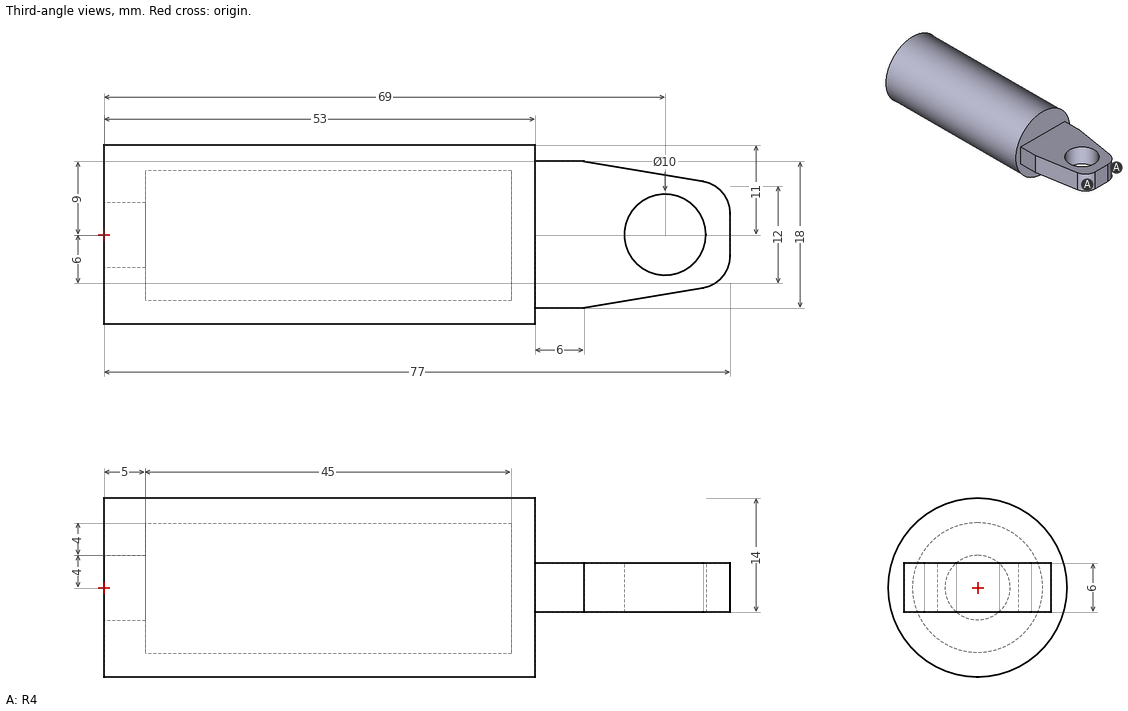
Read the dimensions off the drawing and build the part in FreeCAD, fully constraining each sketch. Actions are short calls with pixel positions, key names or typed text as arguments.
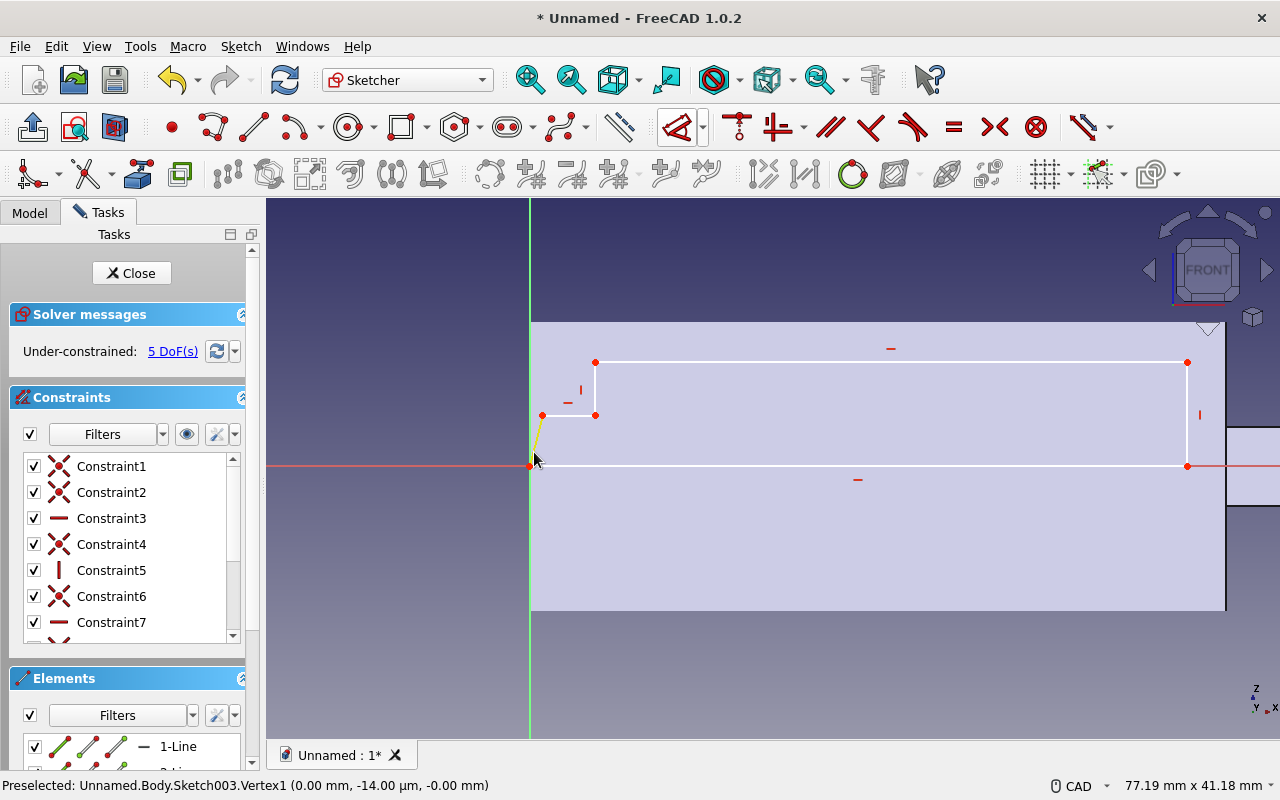
click(534, 451)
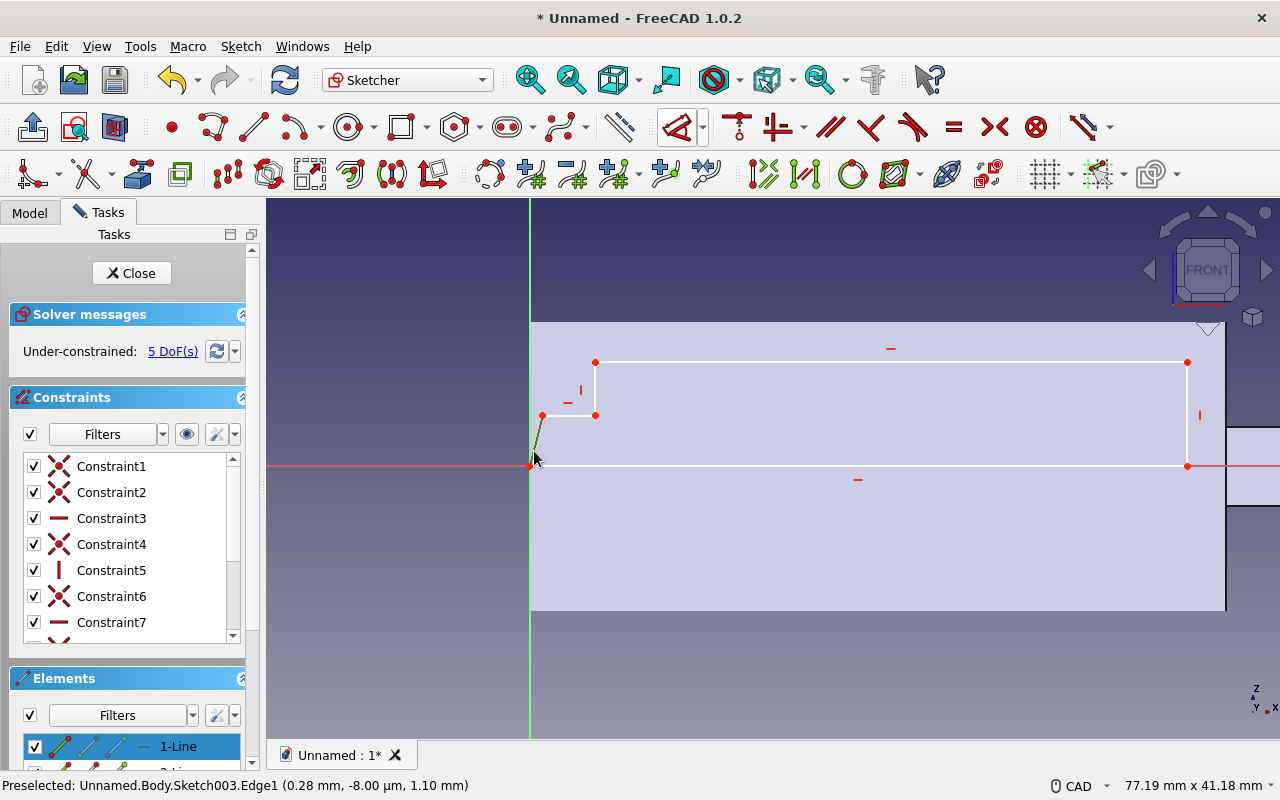
key(v)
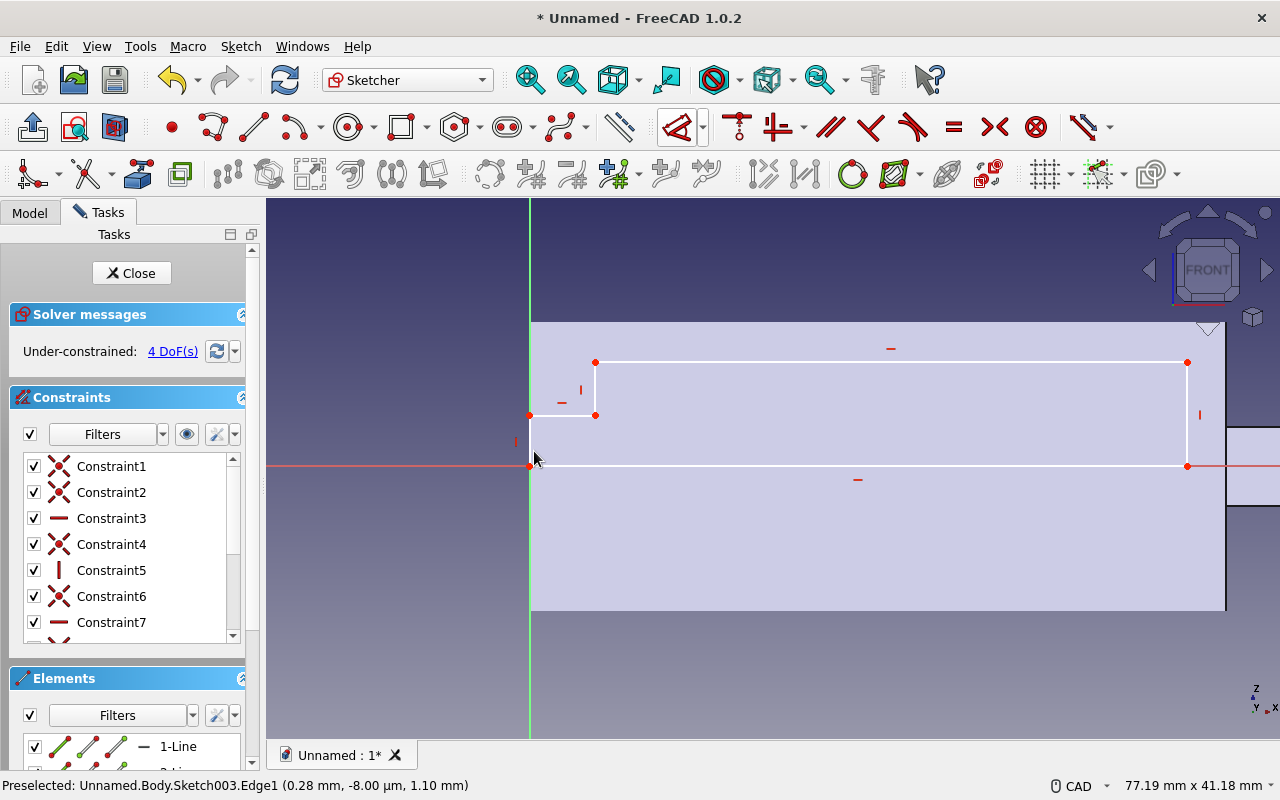
click(530, 451)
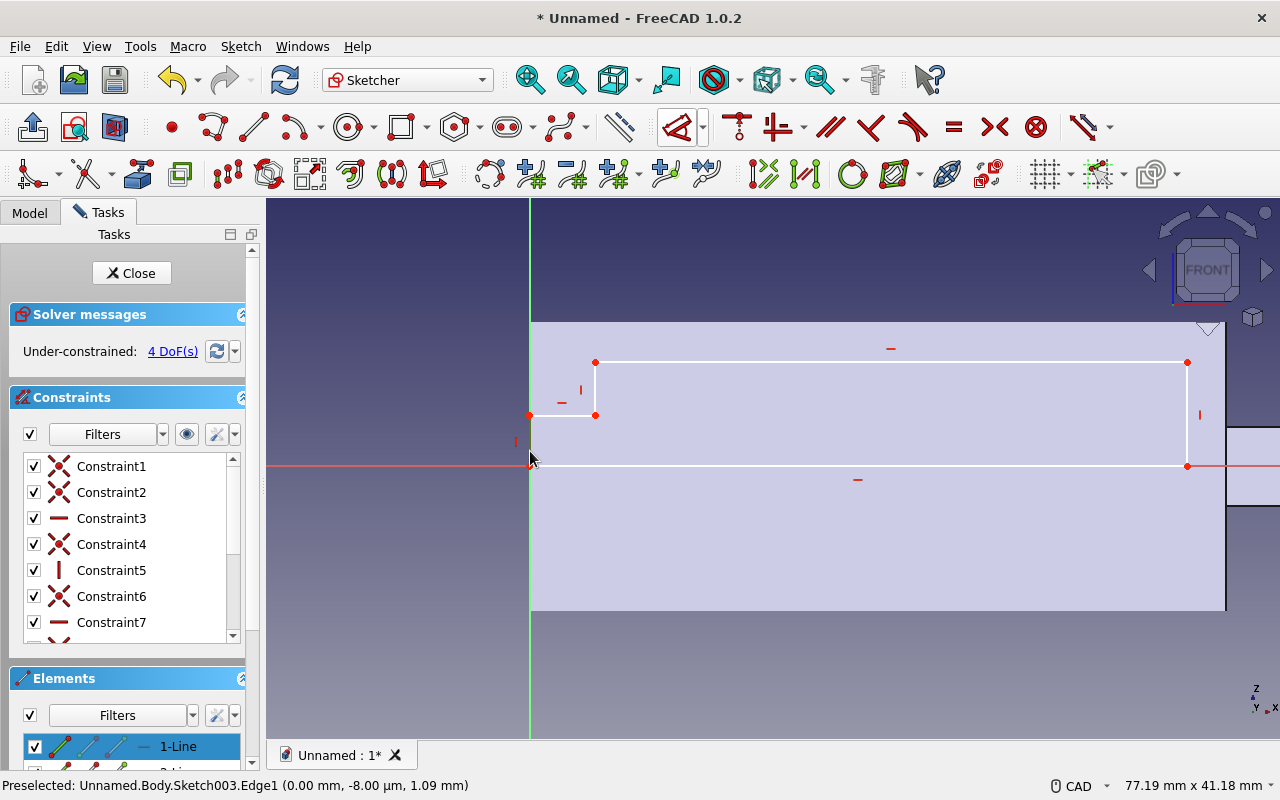
key(i)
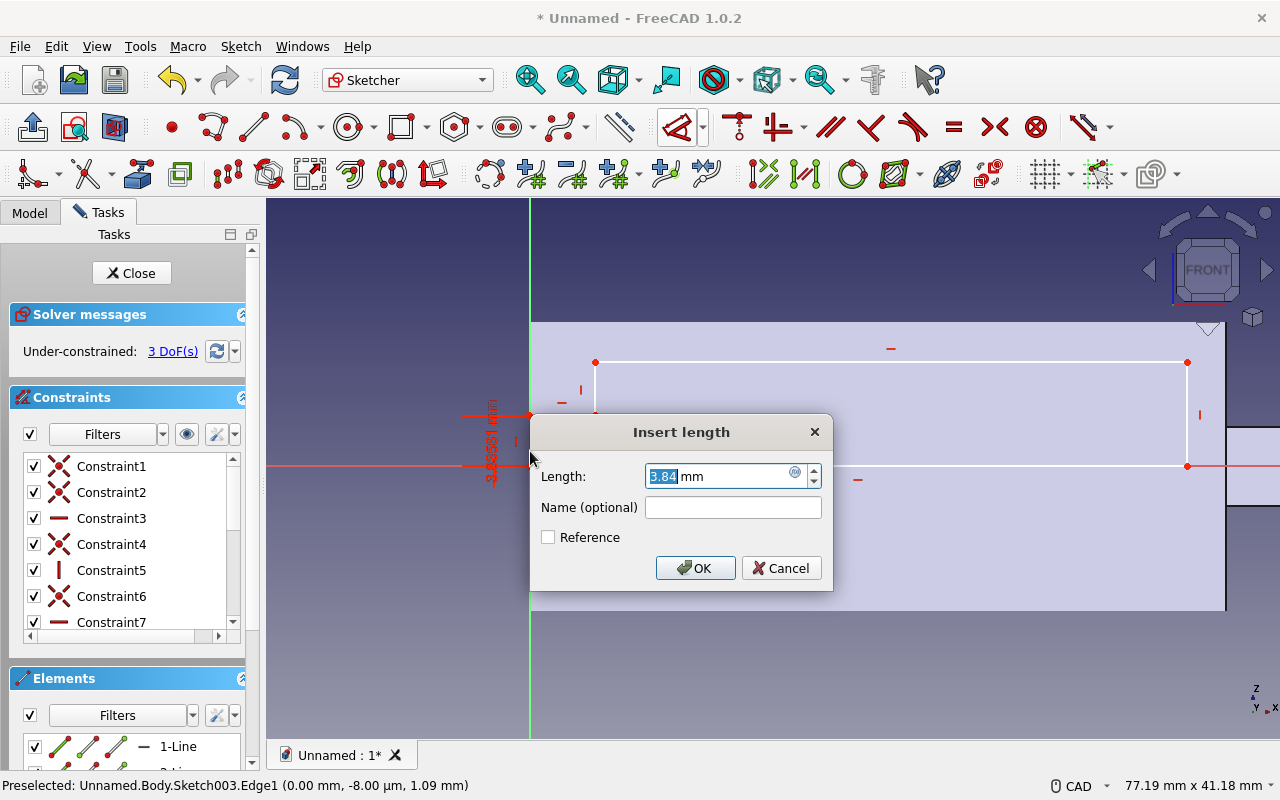
text(4)
key(Return)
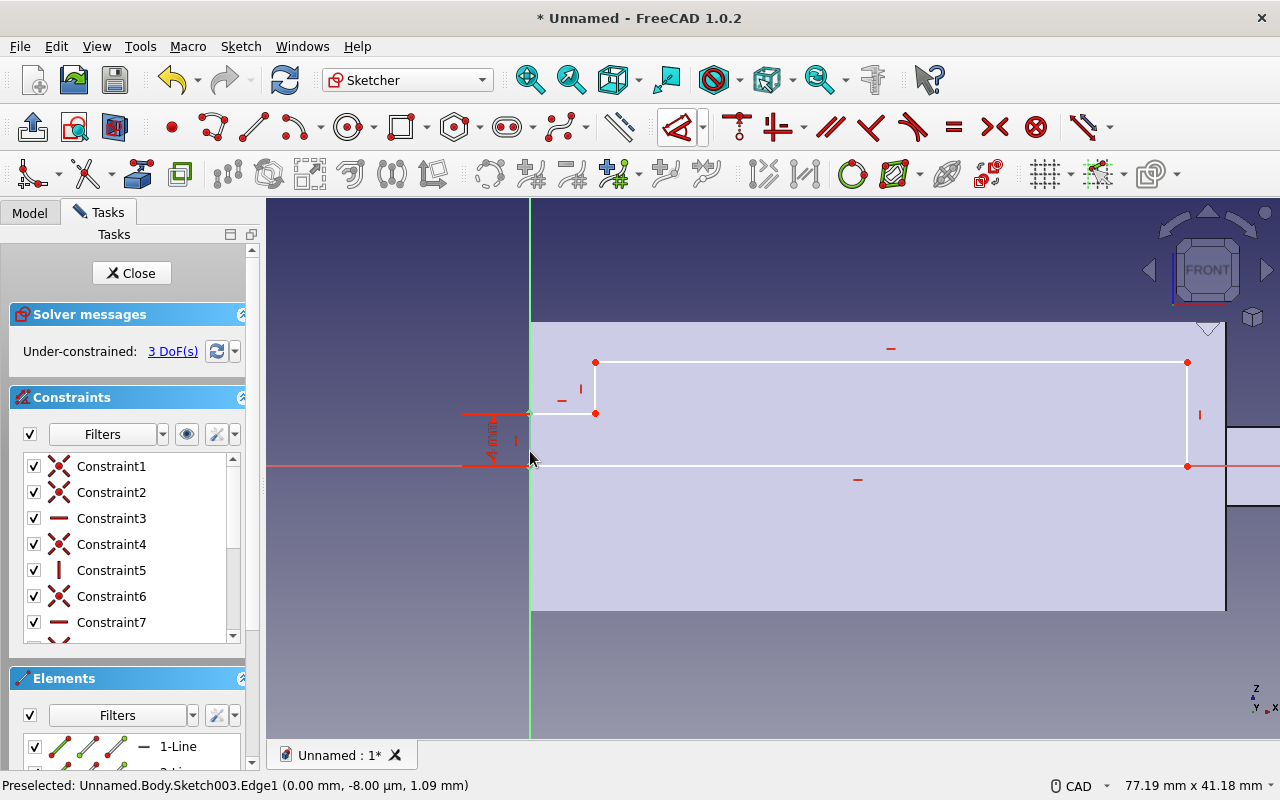
click(549, 414)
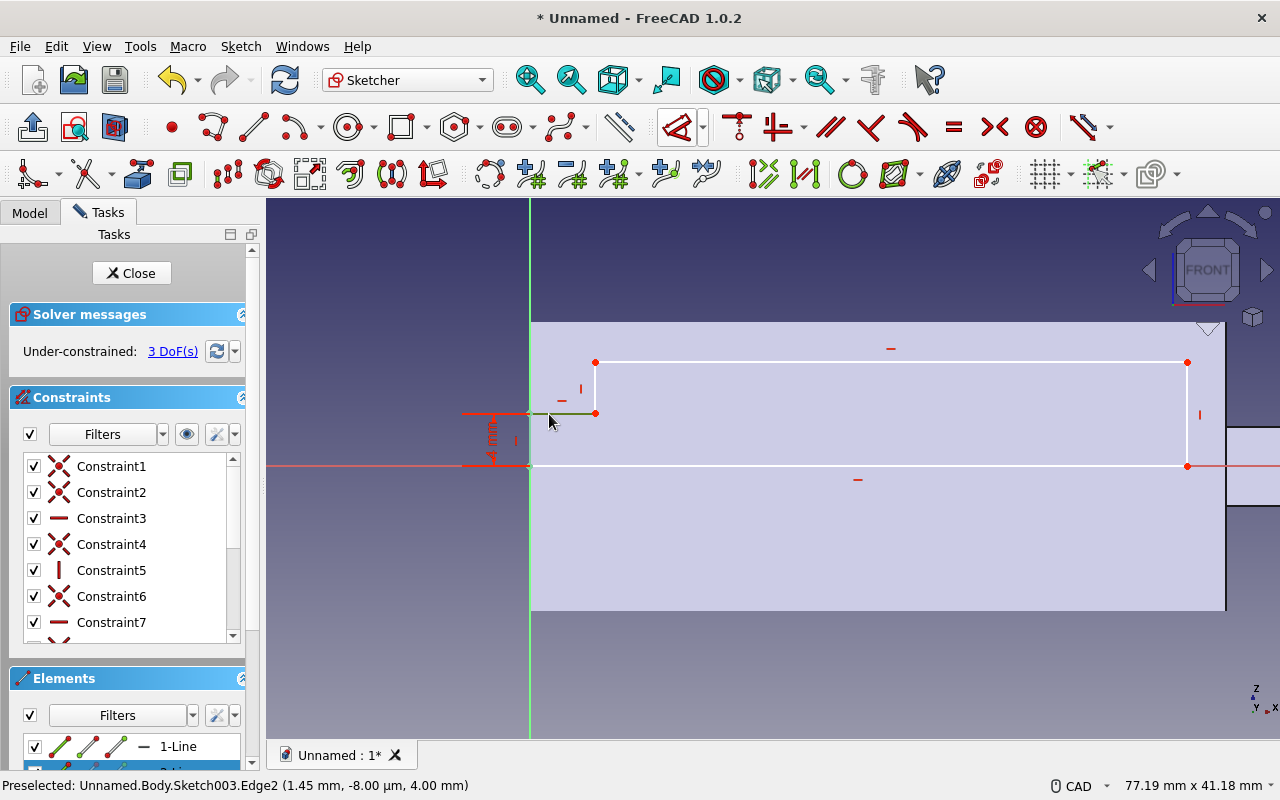
key(l)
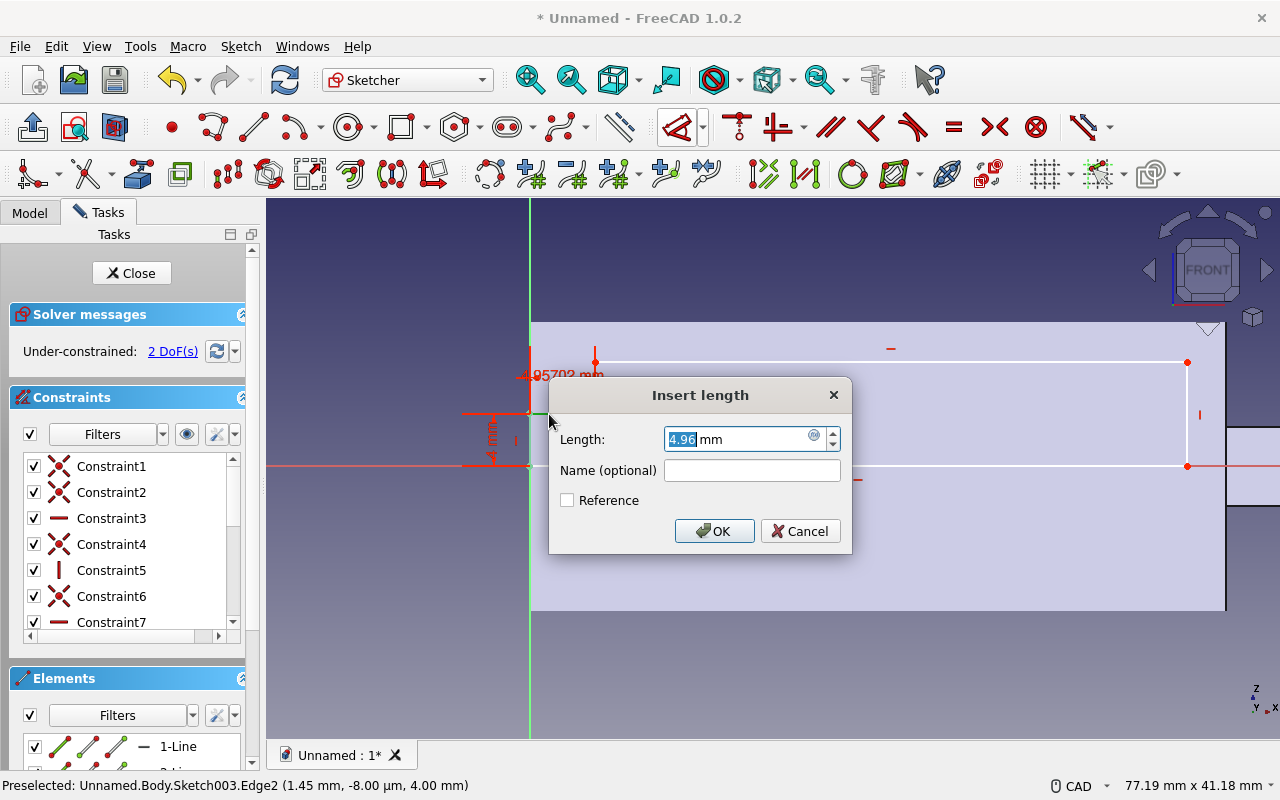
text(5)
key(Return)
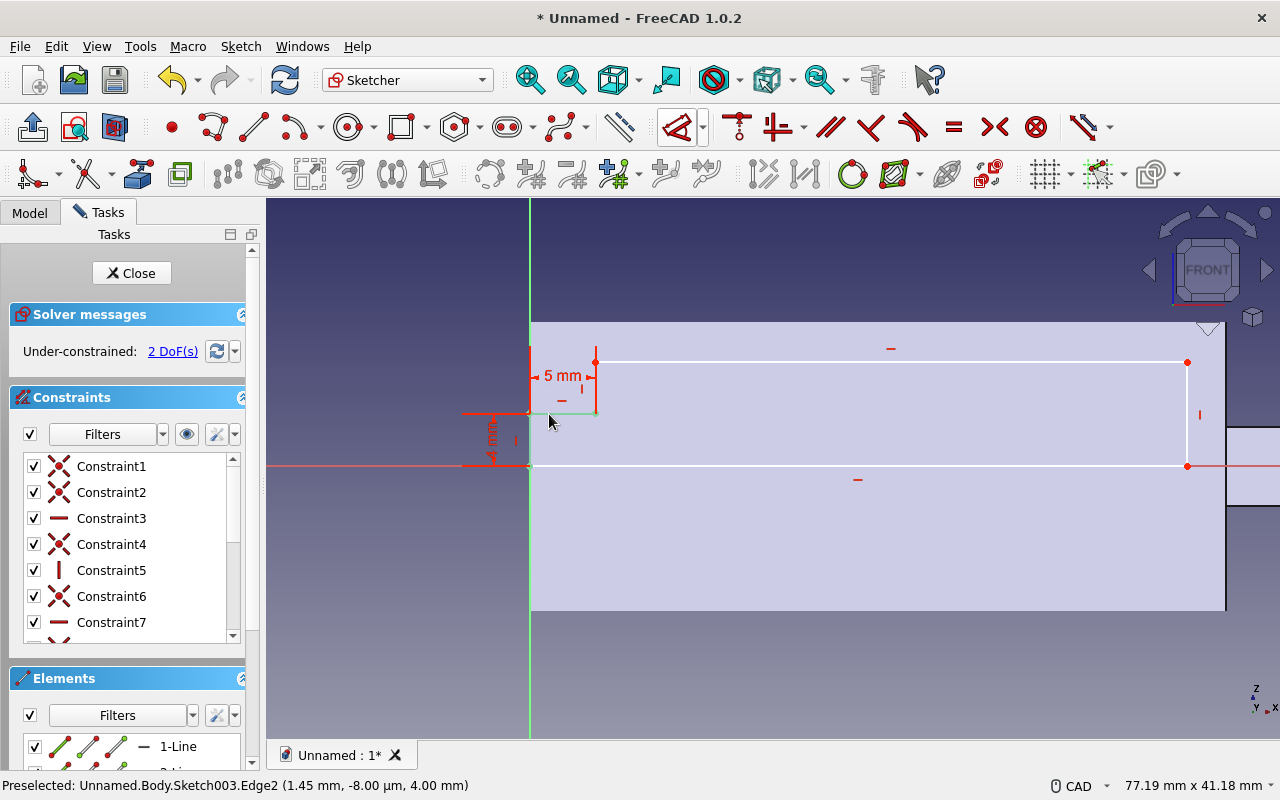
click(596, 398)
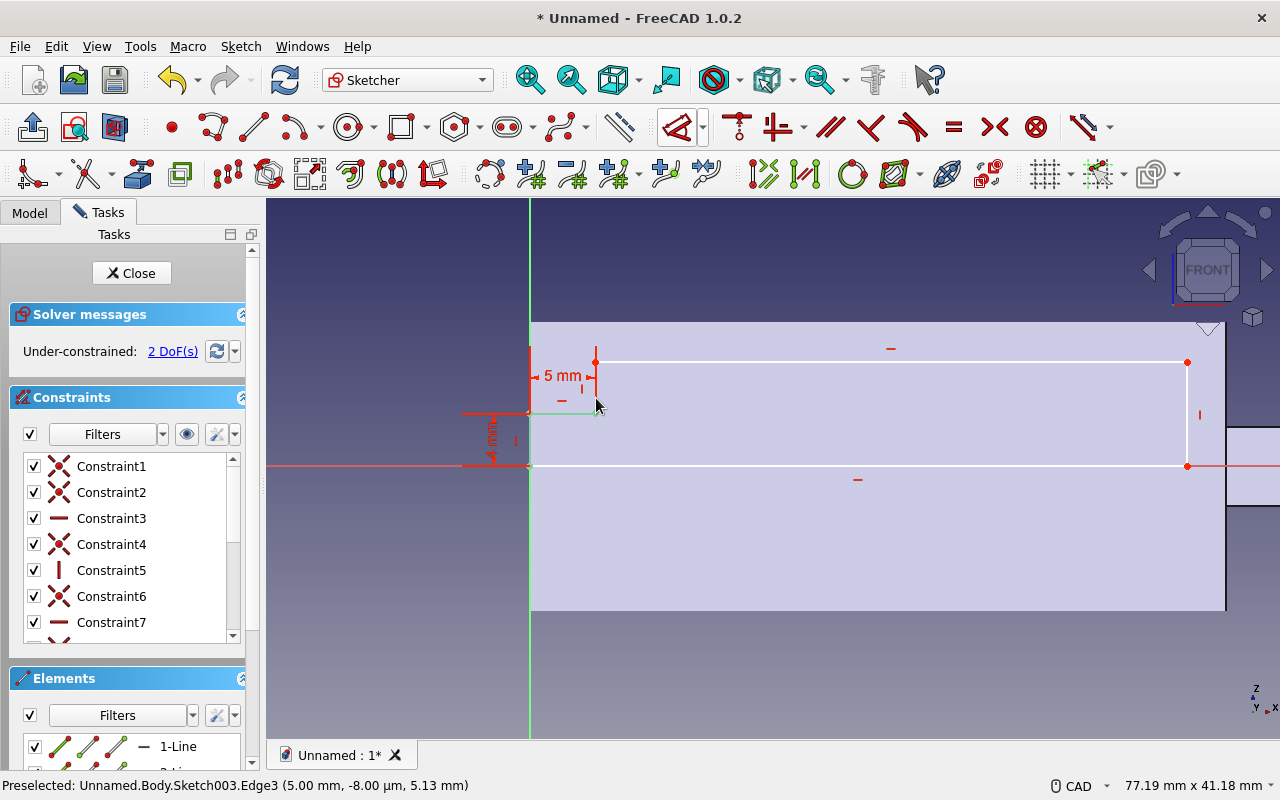
key(i)